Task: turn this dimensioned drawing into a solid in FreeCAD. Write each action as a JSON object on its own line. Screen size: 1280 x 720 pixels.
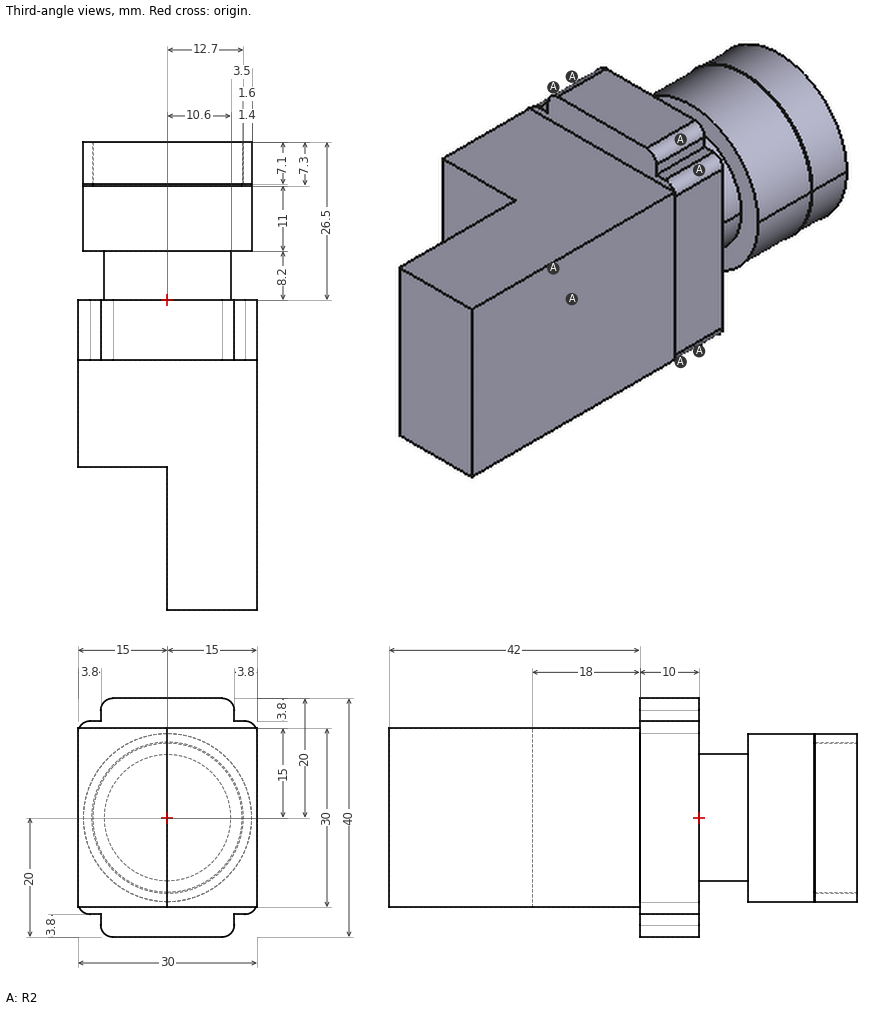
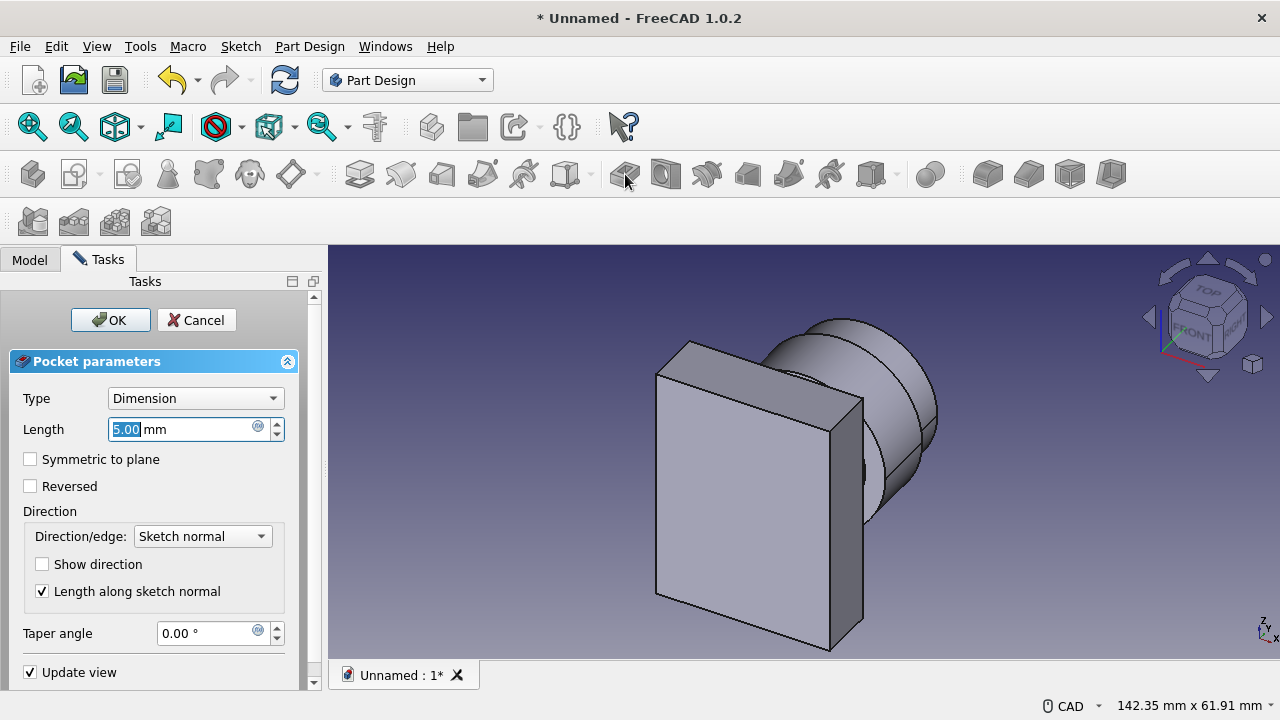
{"action": "type", "text": "10"}
{"action": "key", "text": "Tab"}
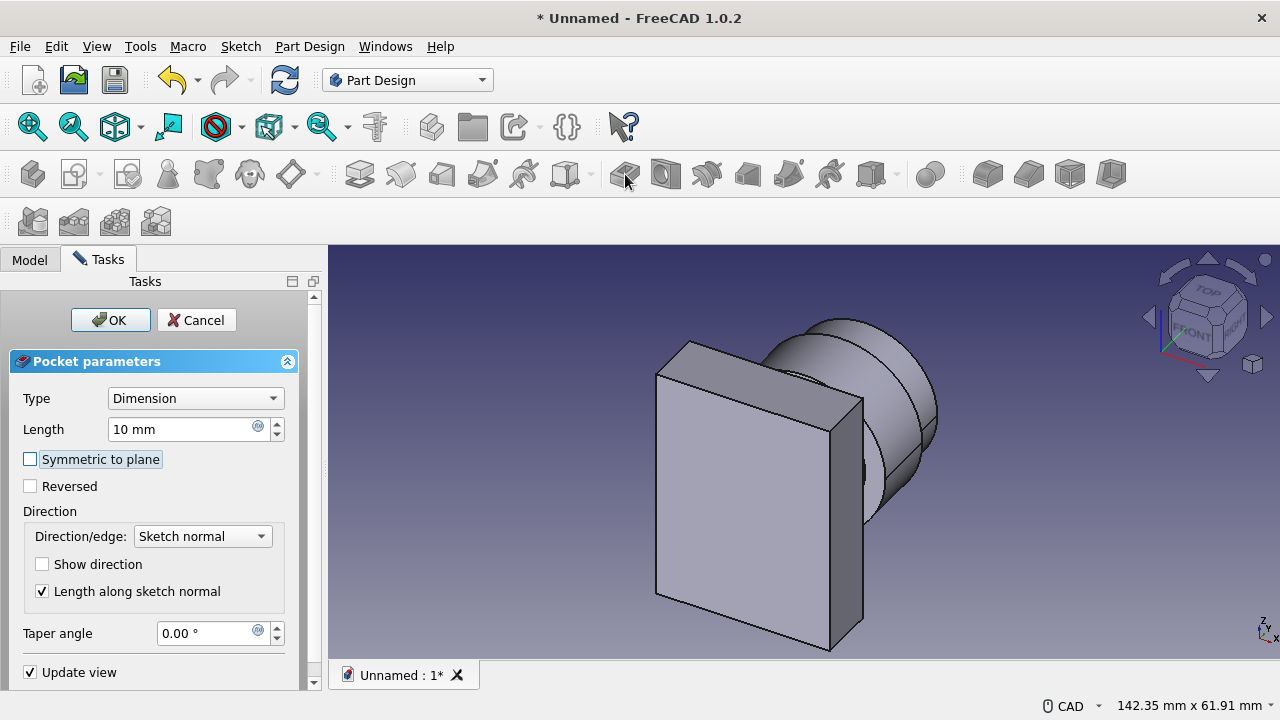
{"action": "left_click", "coordinate": [31, 486]}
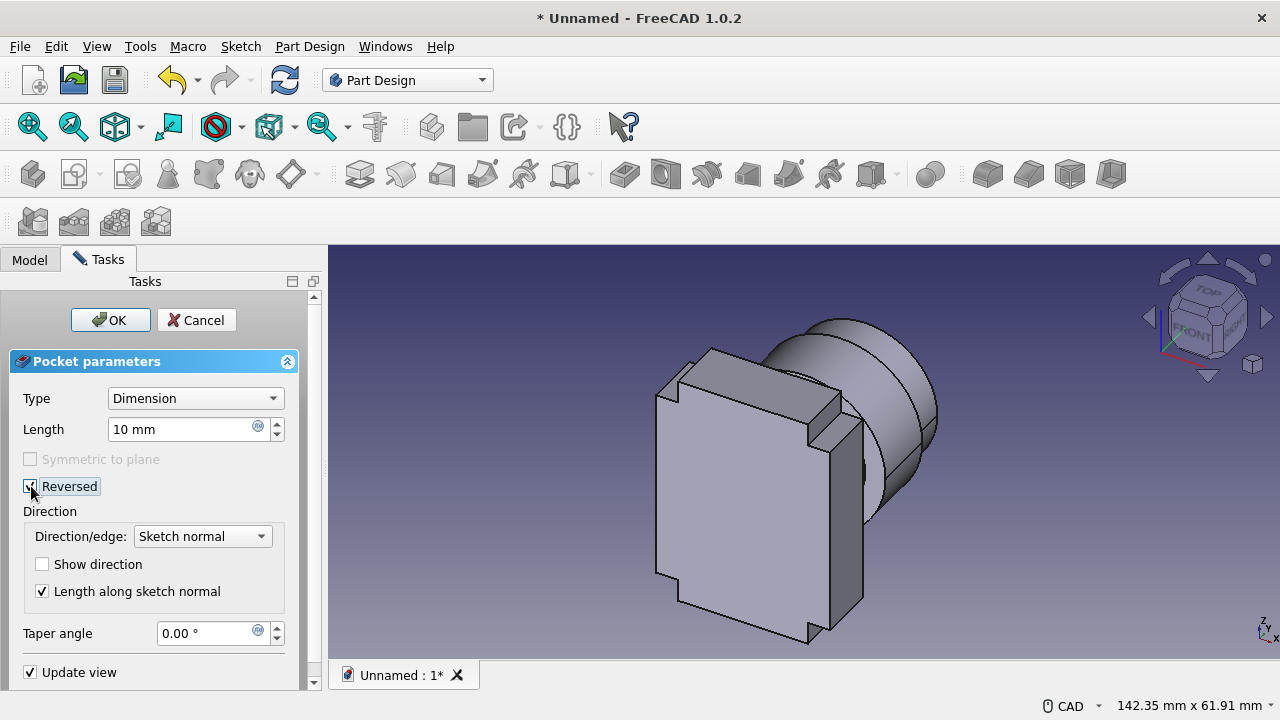
{"action": "left_click", "coordinate": [111, 320]}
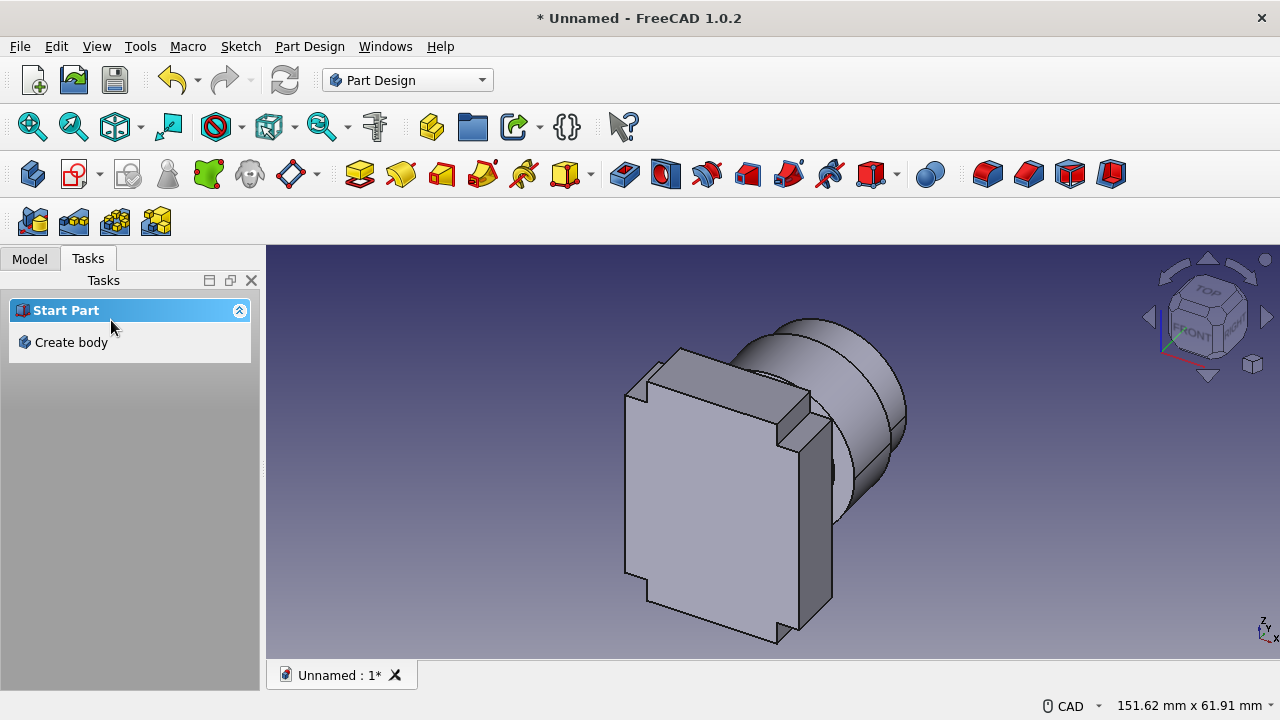
{"action": "left_click", "coordinate": [816, 435]}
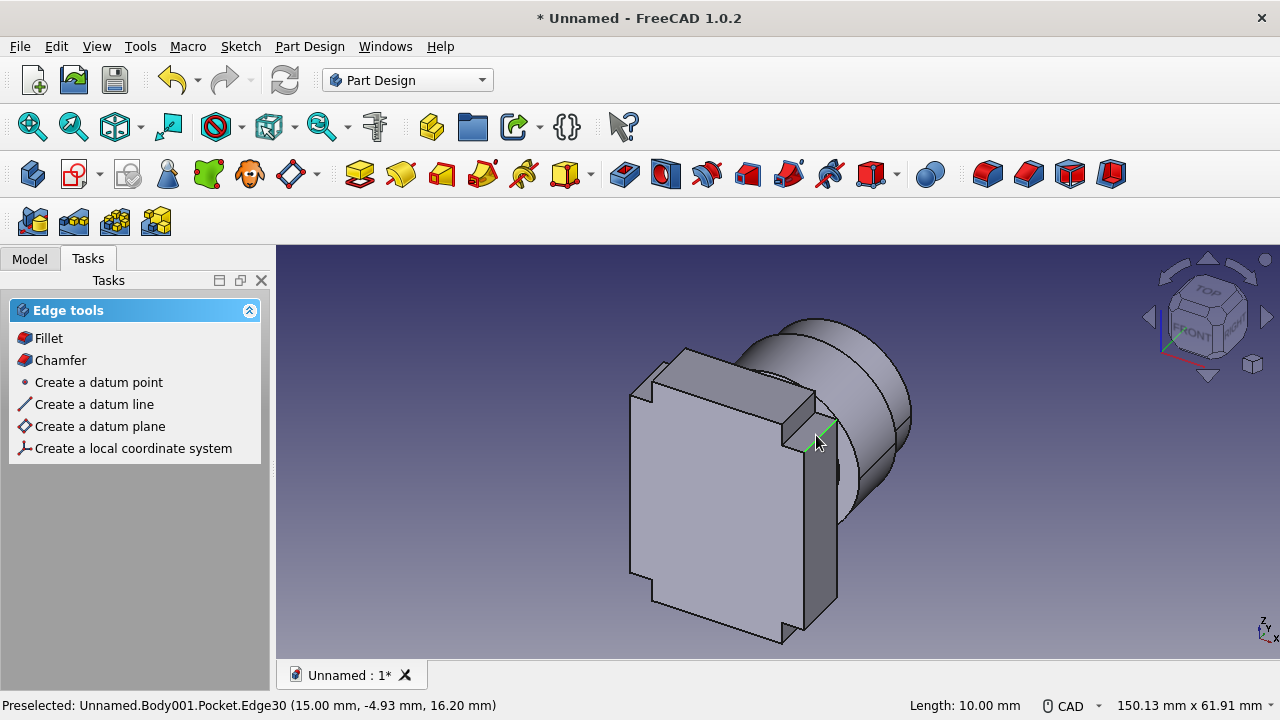
{"action": "left_click", "coordinate": [799, 407], "text": "ctrl"}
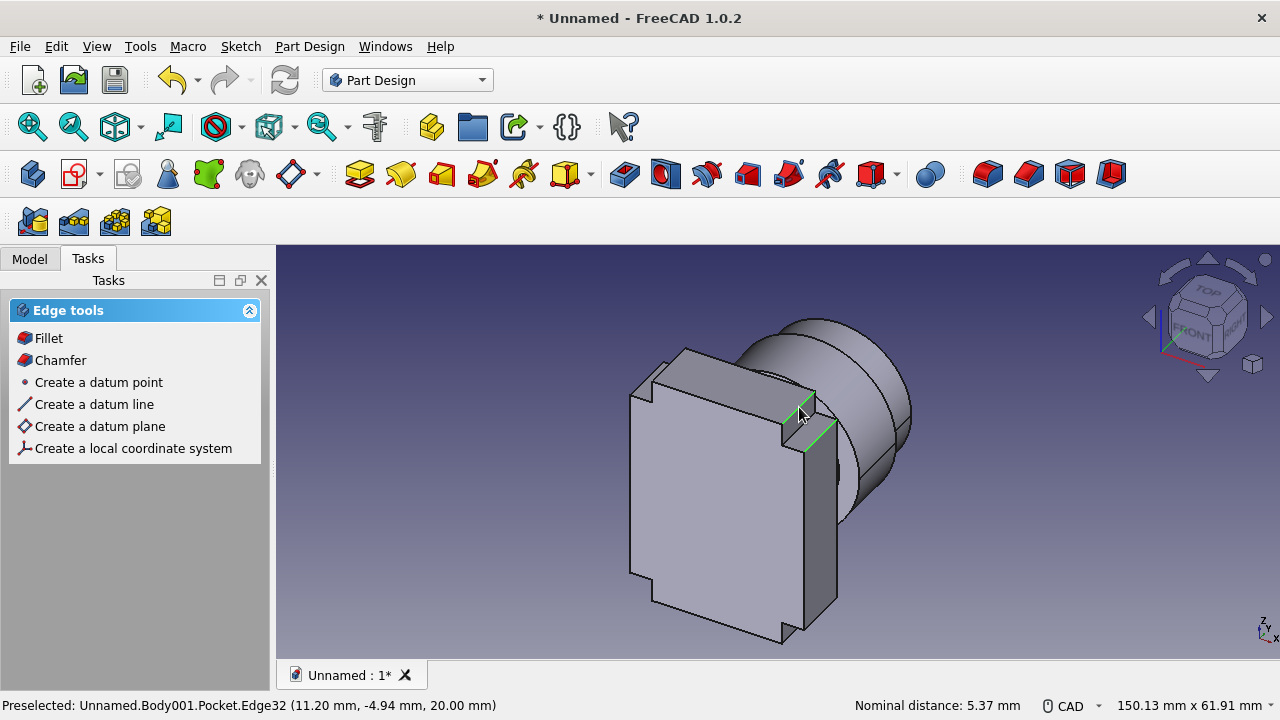
{"action": "key", "text": "0"}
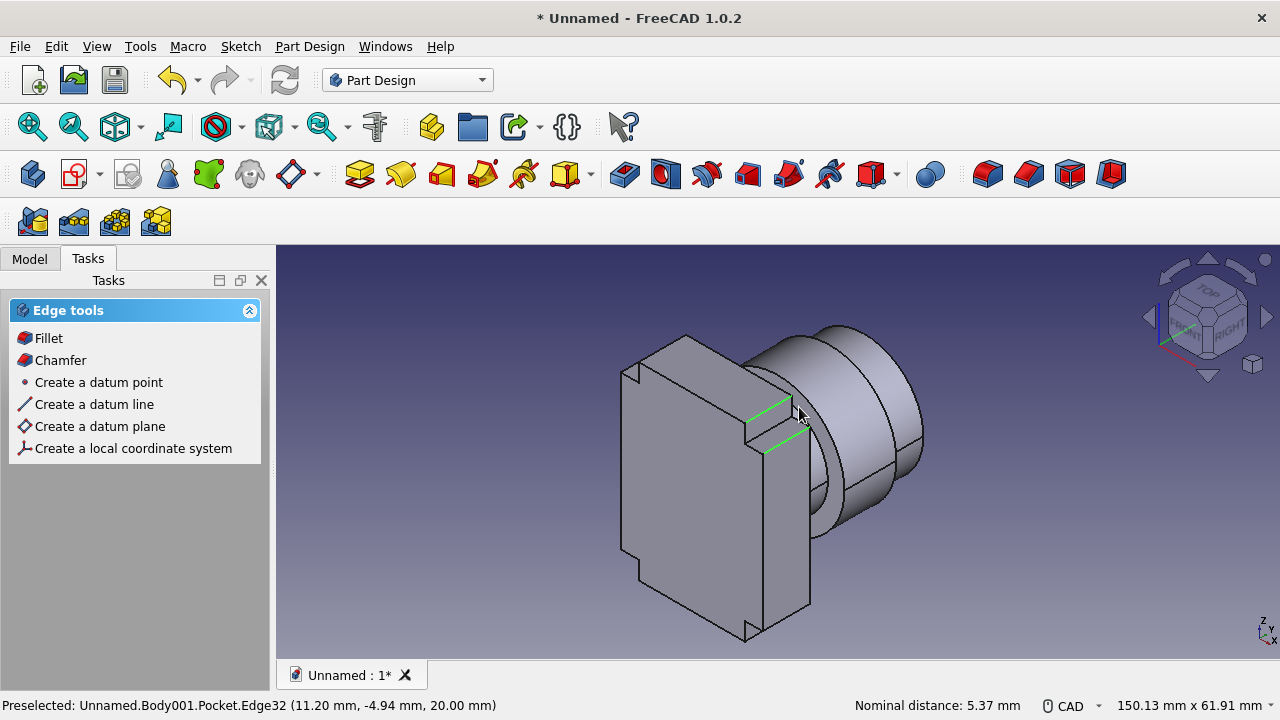
{"action": "key", "text": "2"}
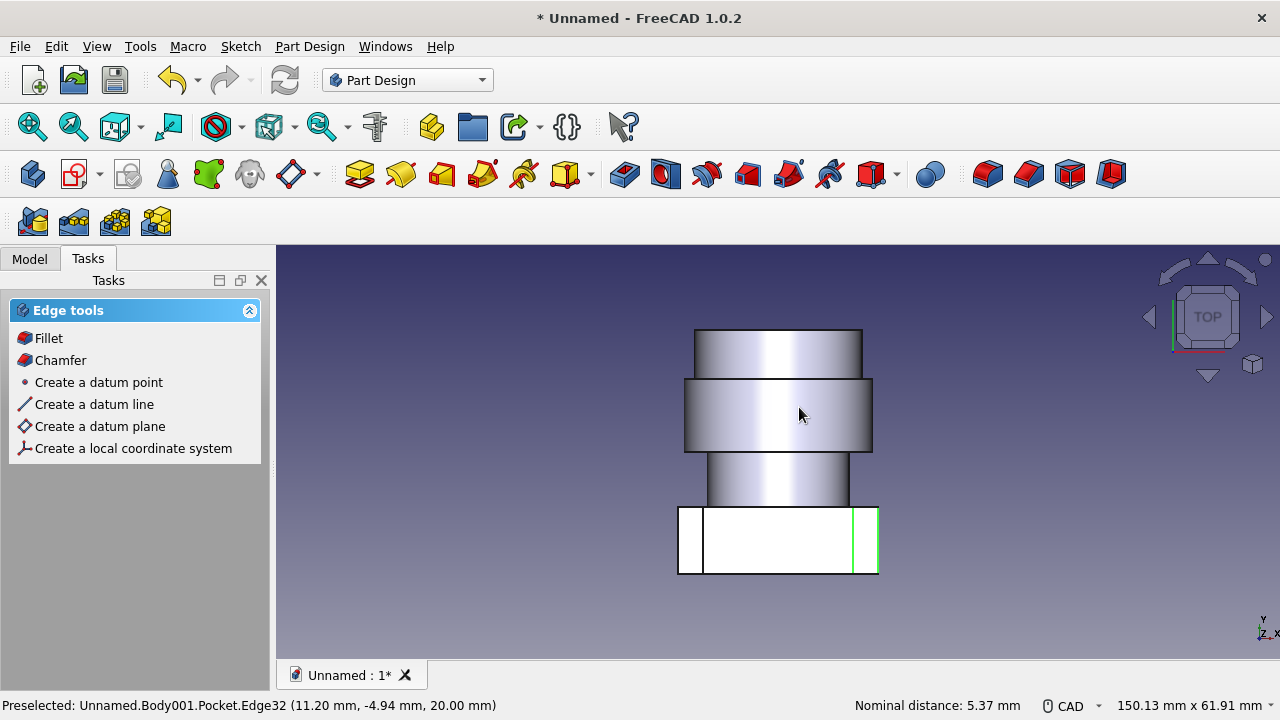
{"action": "key", "text": "v f"}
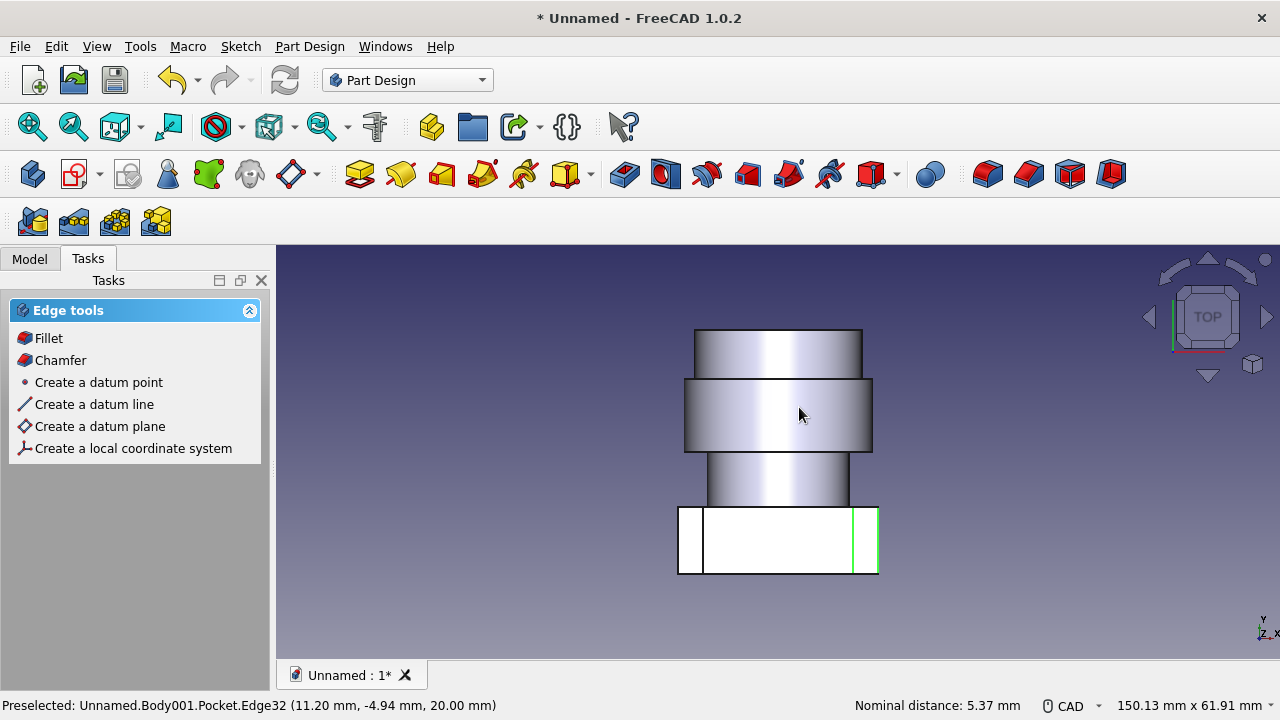
{"action": "left_click", "coordinate": [703, 540], "text": "ctrl"}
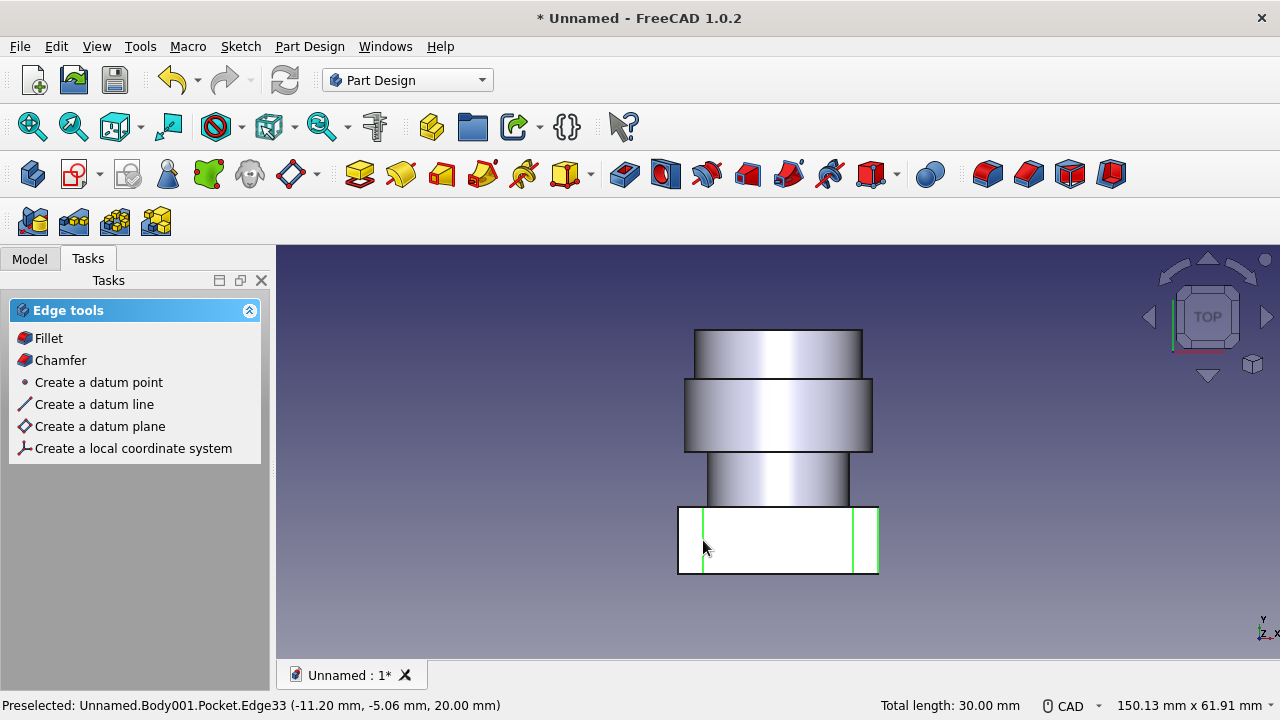
{"action": "left_click", "coordinate": [678, 540], "text": "ctrl"}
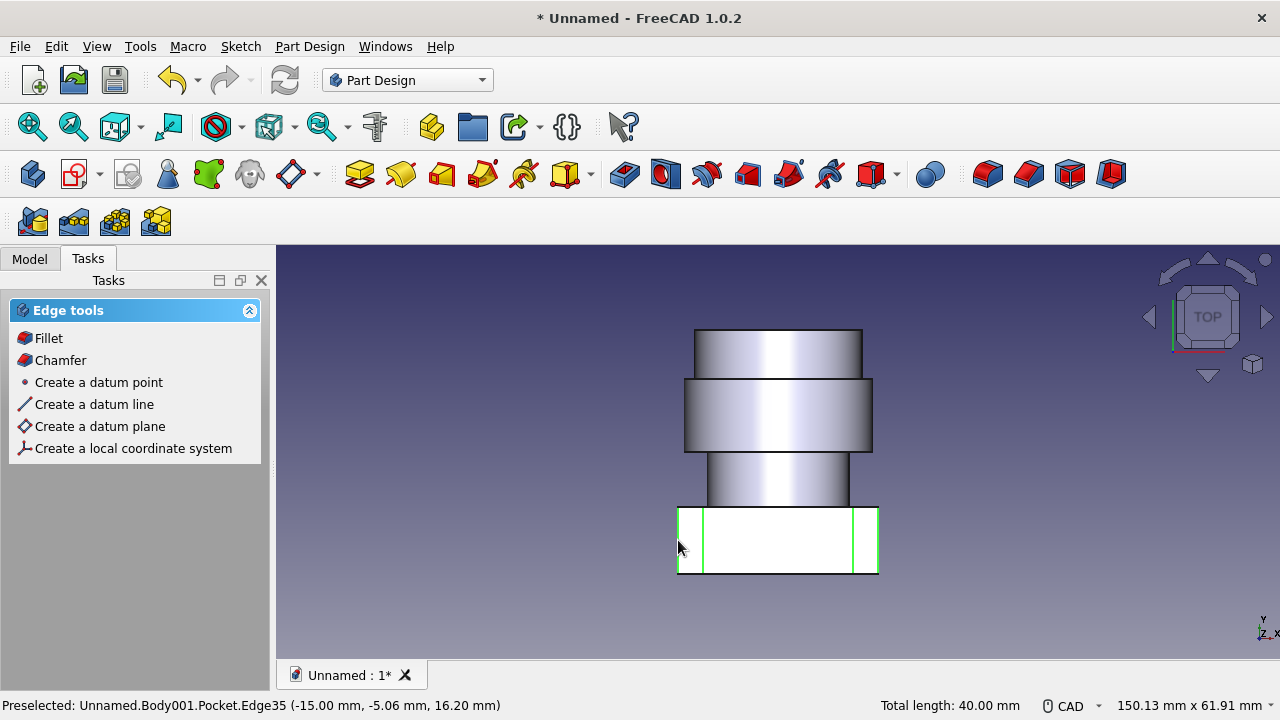
{"action": "key", "text": "1"}